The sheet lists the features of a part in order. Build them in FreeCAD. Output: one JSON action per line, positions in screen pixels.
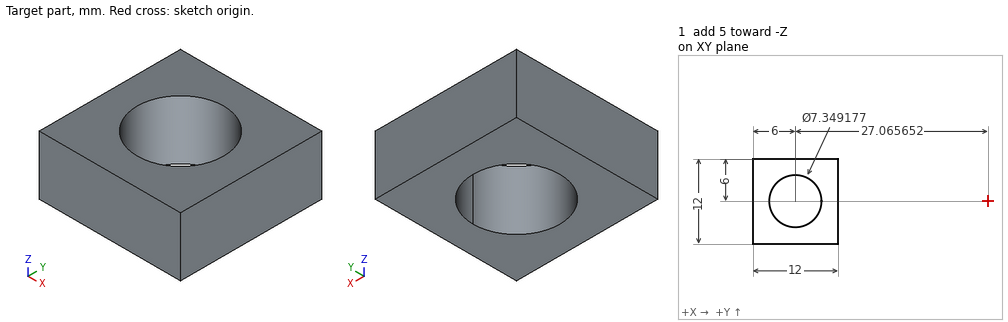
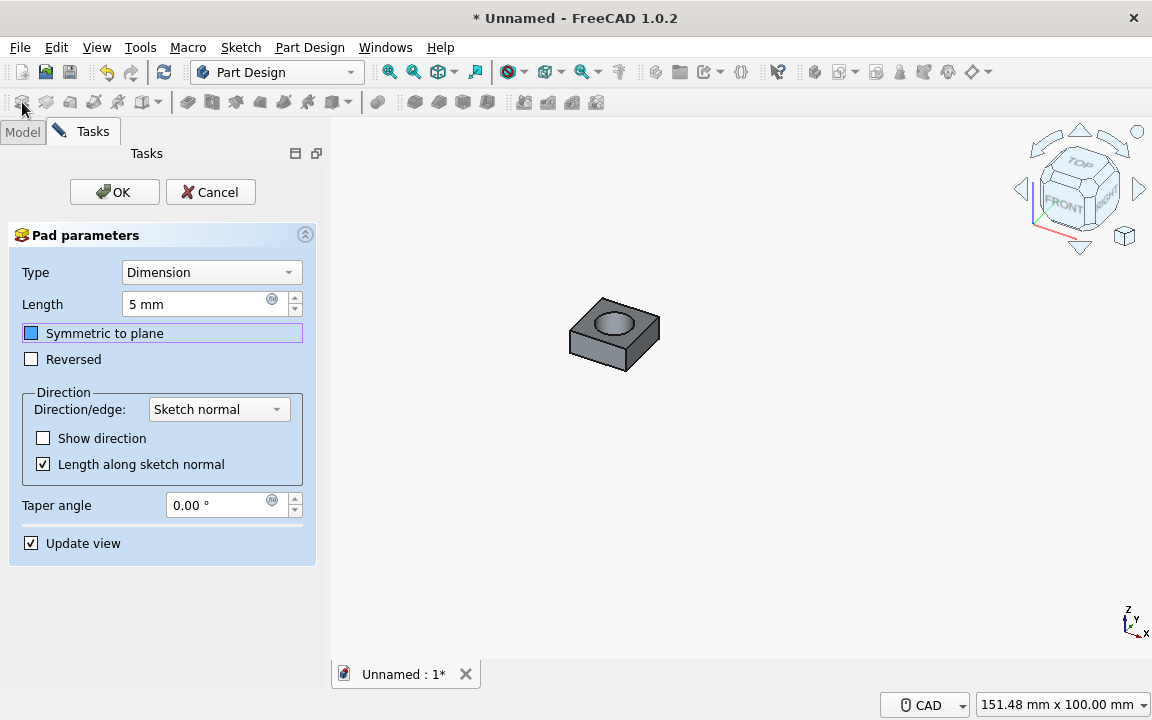
{"action": "left_click", "coordinate": [30, 359]}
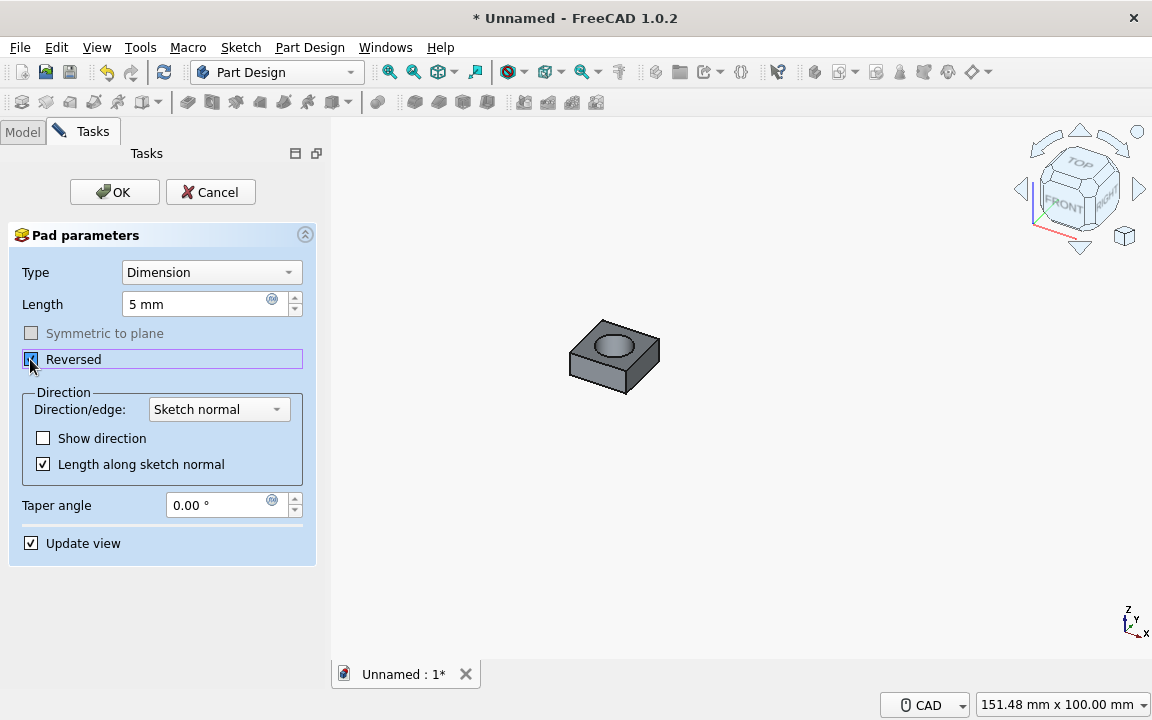
{"action": "left_click", "coordinate": [115, 192]}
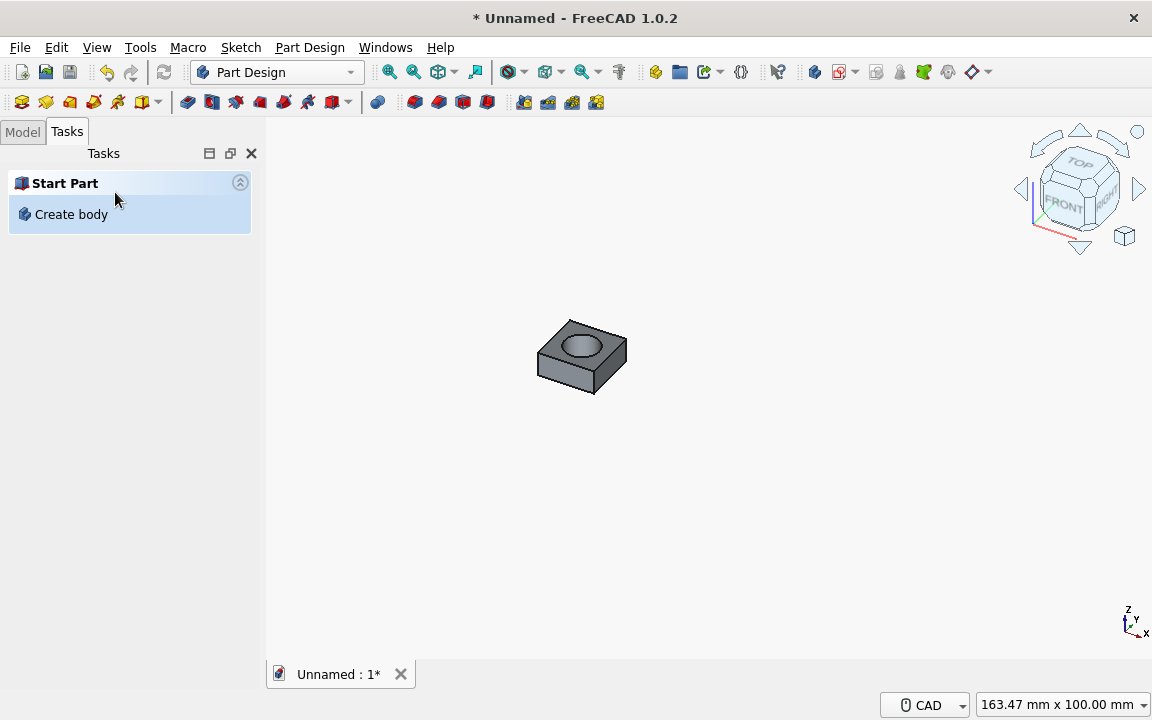
{"action": "key", "text": "0"}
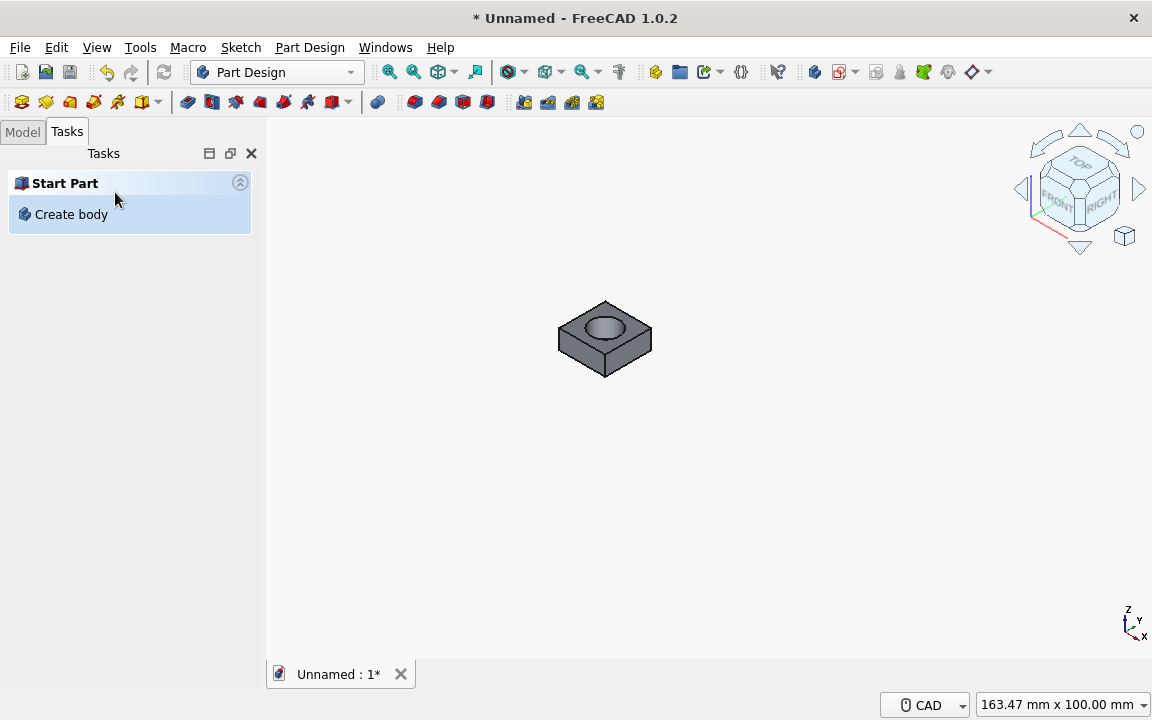
{"action": "key", "text": "v f"}